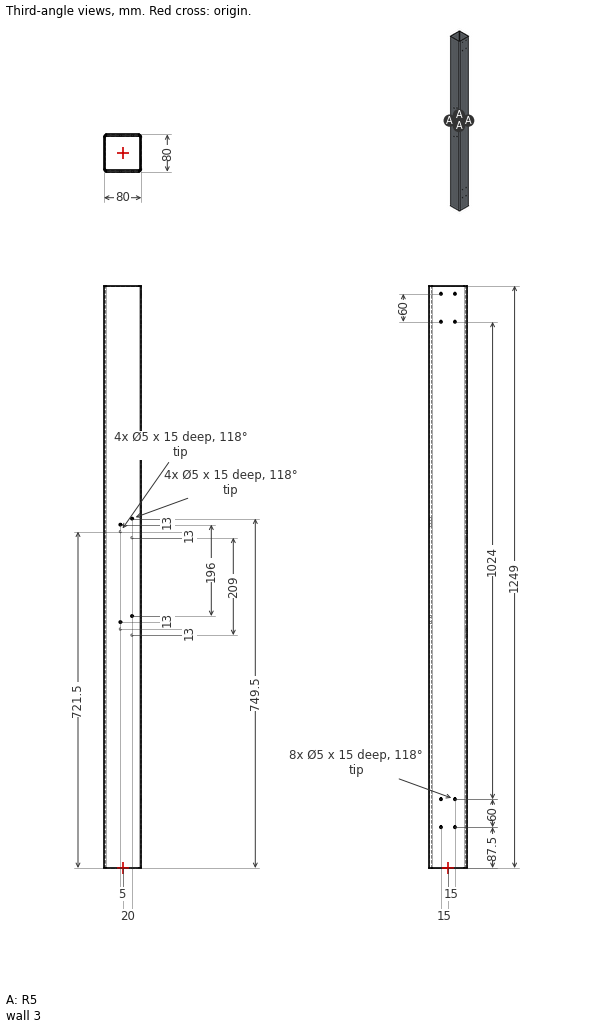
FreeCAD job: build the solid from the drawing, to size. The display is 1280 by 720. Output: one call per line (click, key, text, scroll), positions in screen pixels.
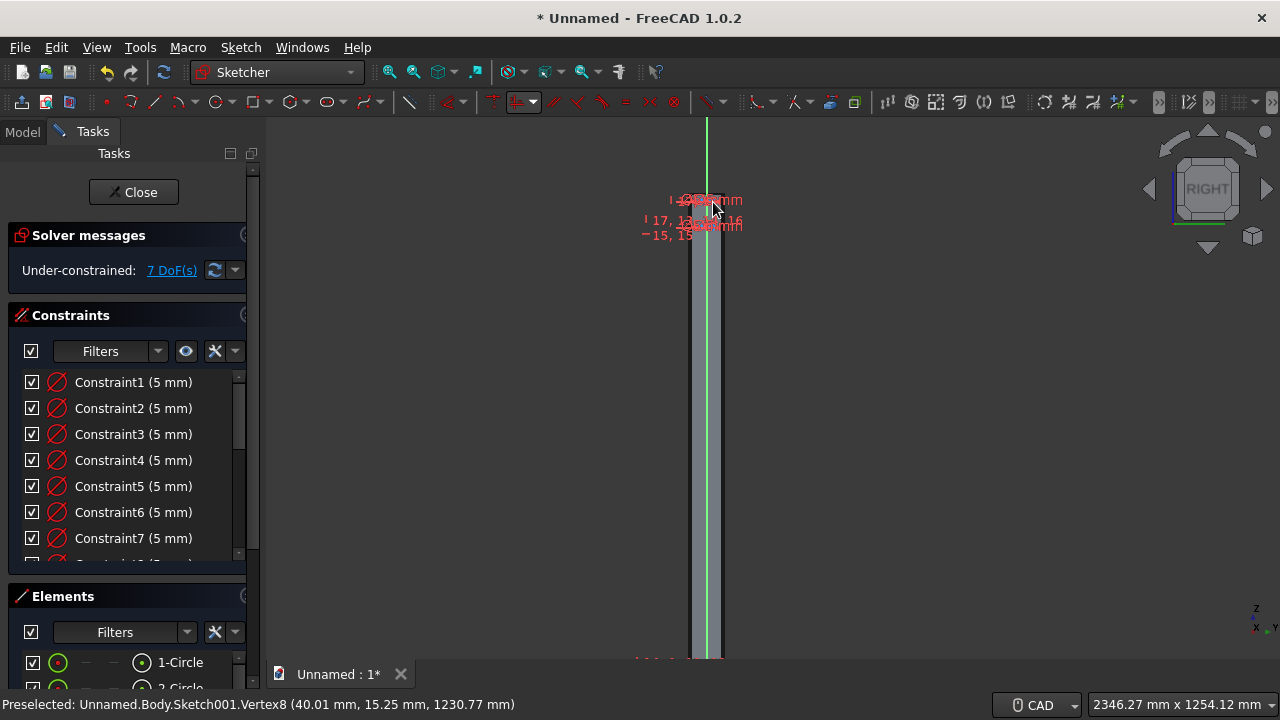
scroll(700, 202, up, 4)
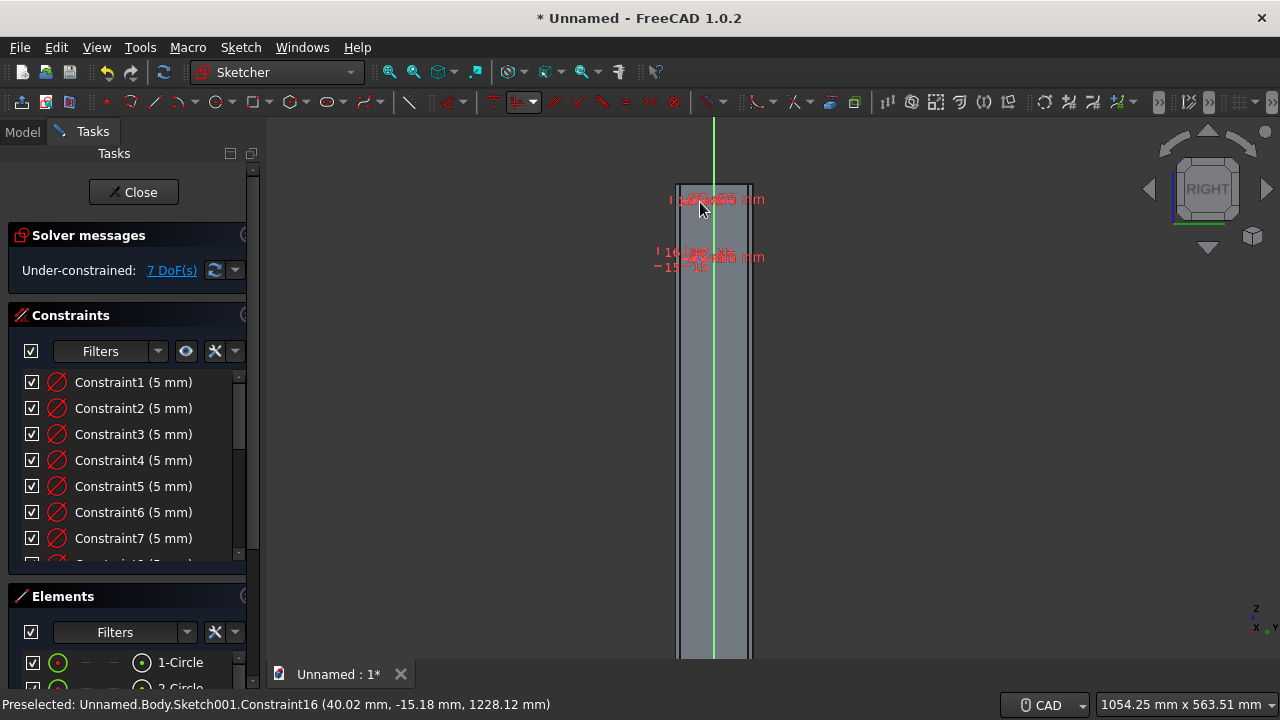
scroll(700, 201, up, 4)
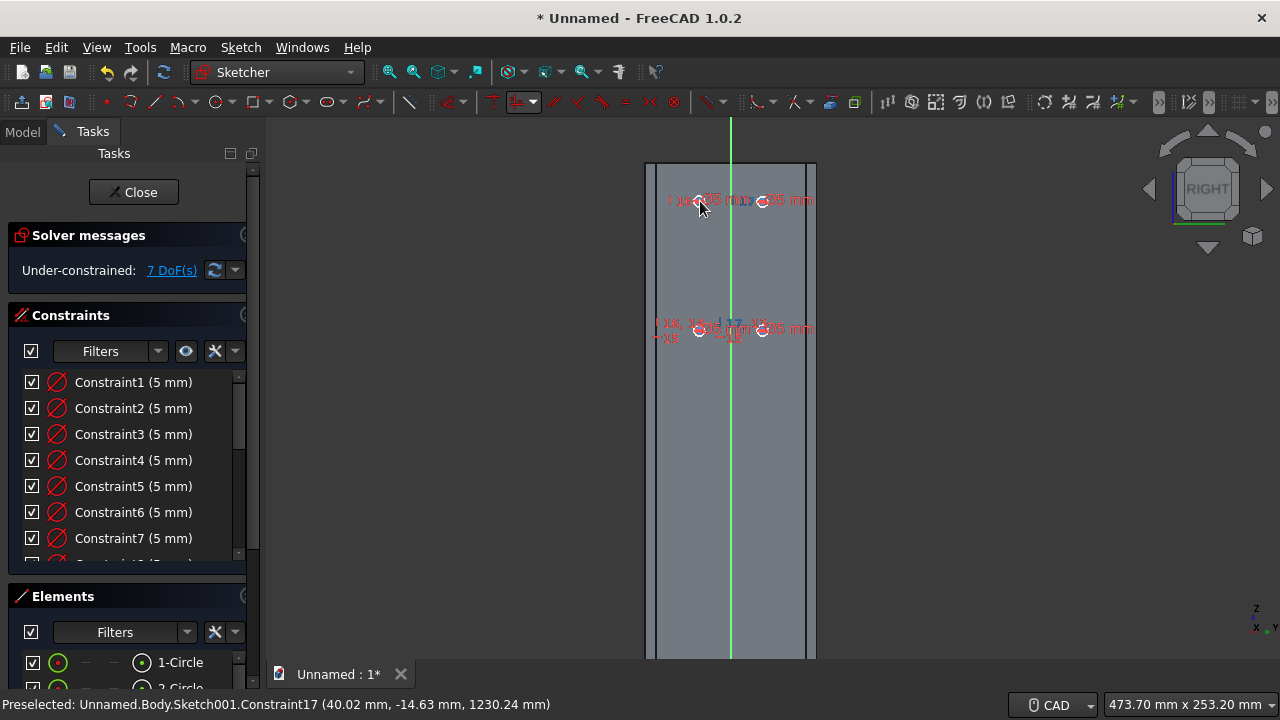
click(699, 201)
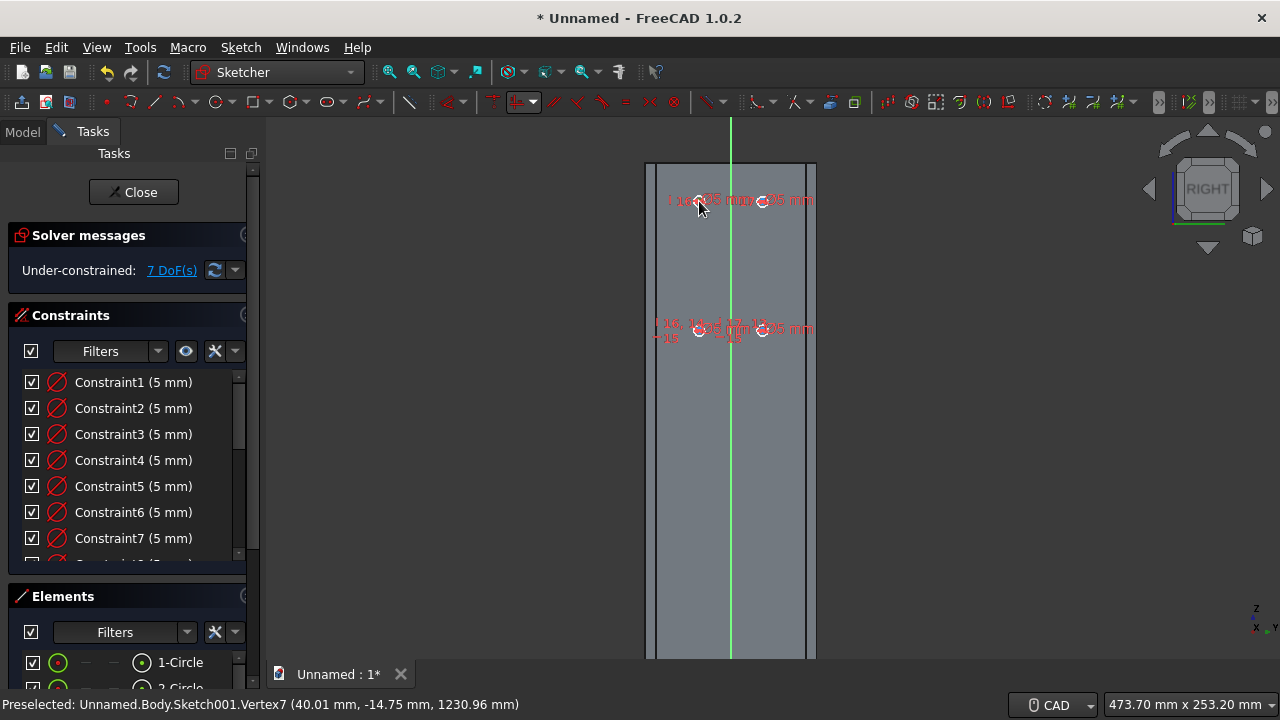
scroll(700, 211, down, 10)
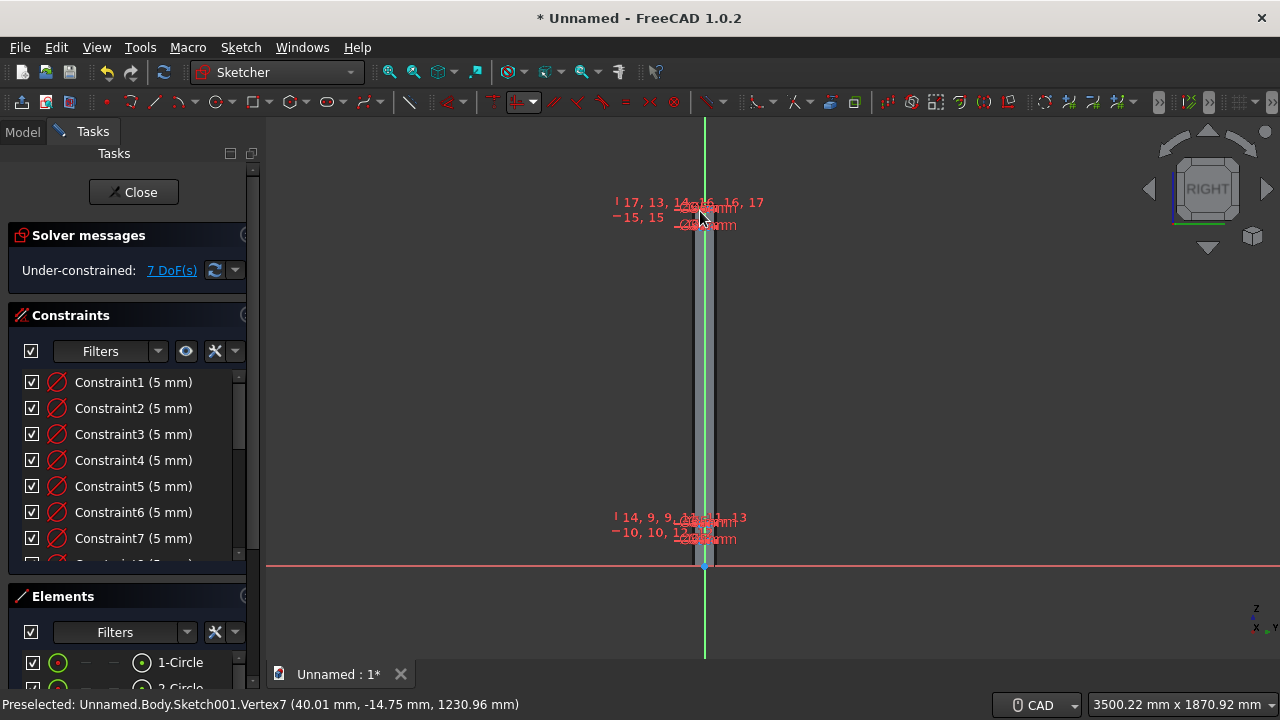
scroll(709, 210, up, 2)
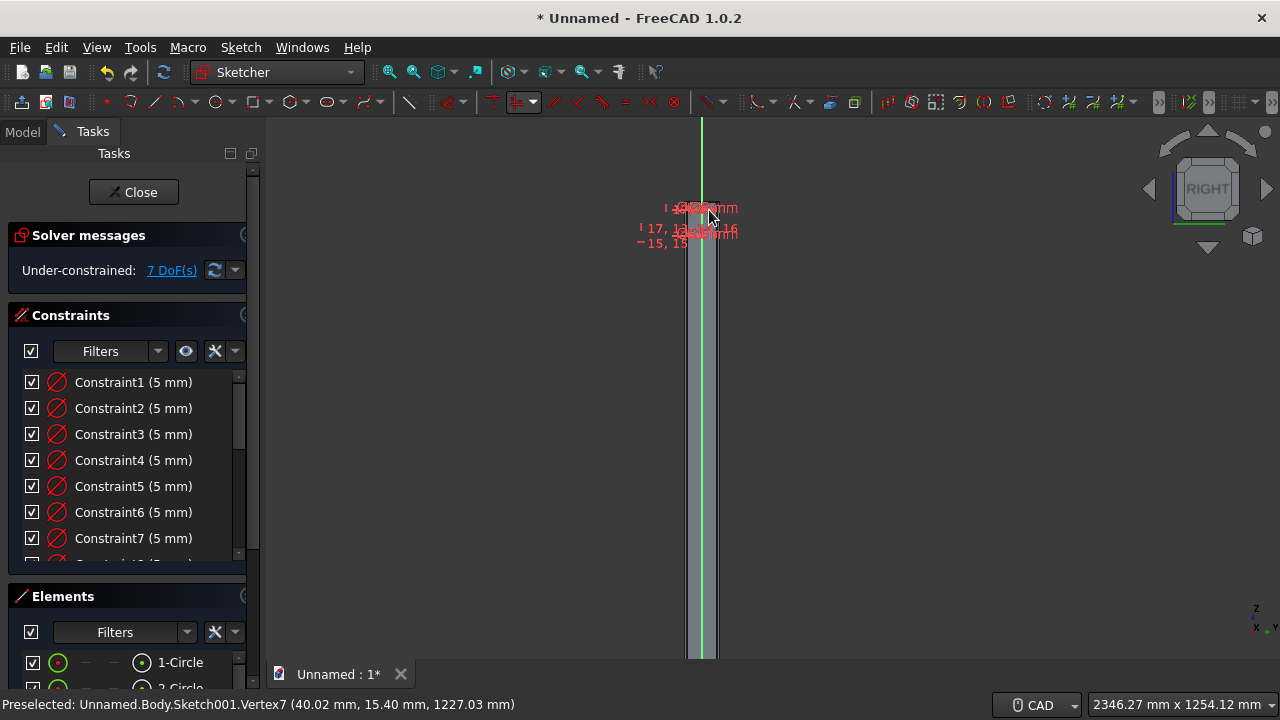
scroll(709, 210, up, 4)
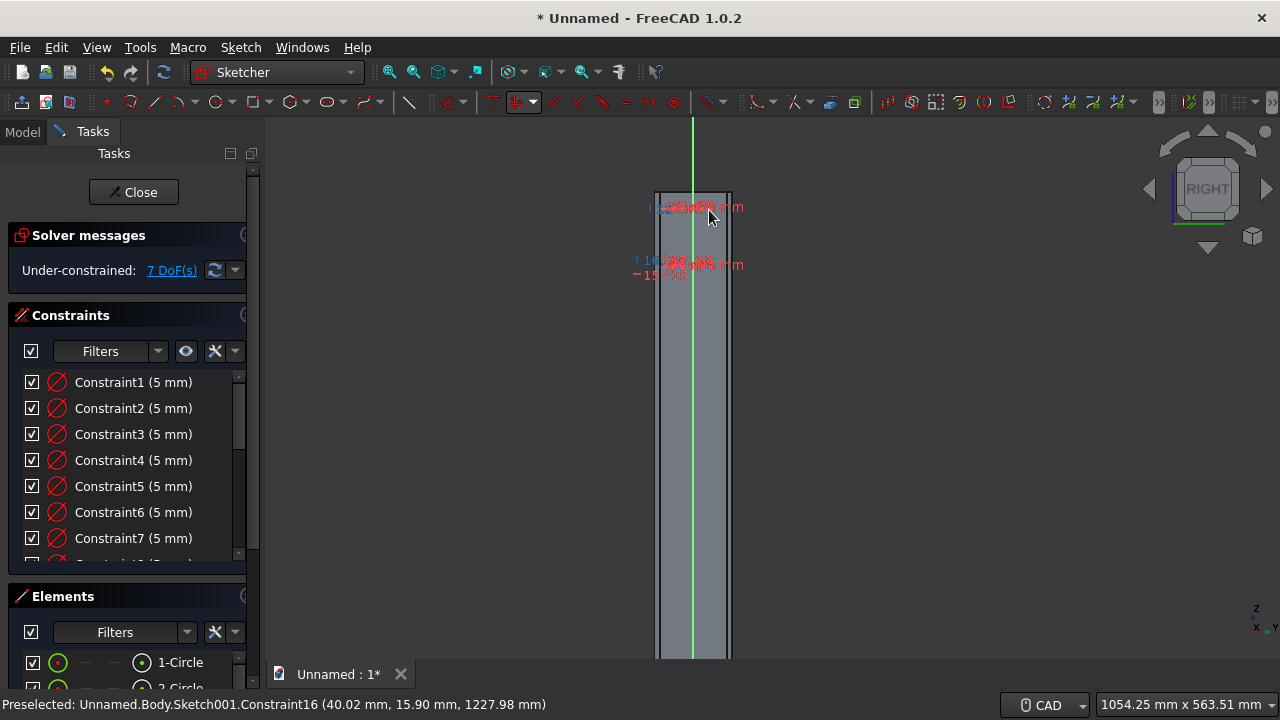
click(707, 209)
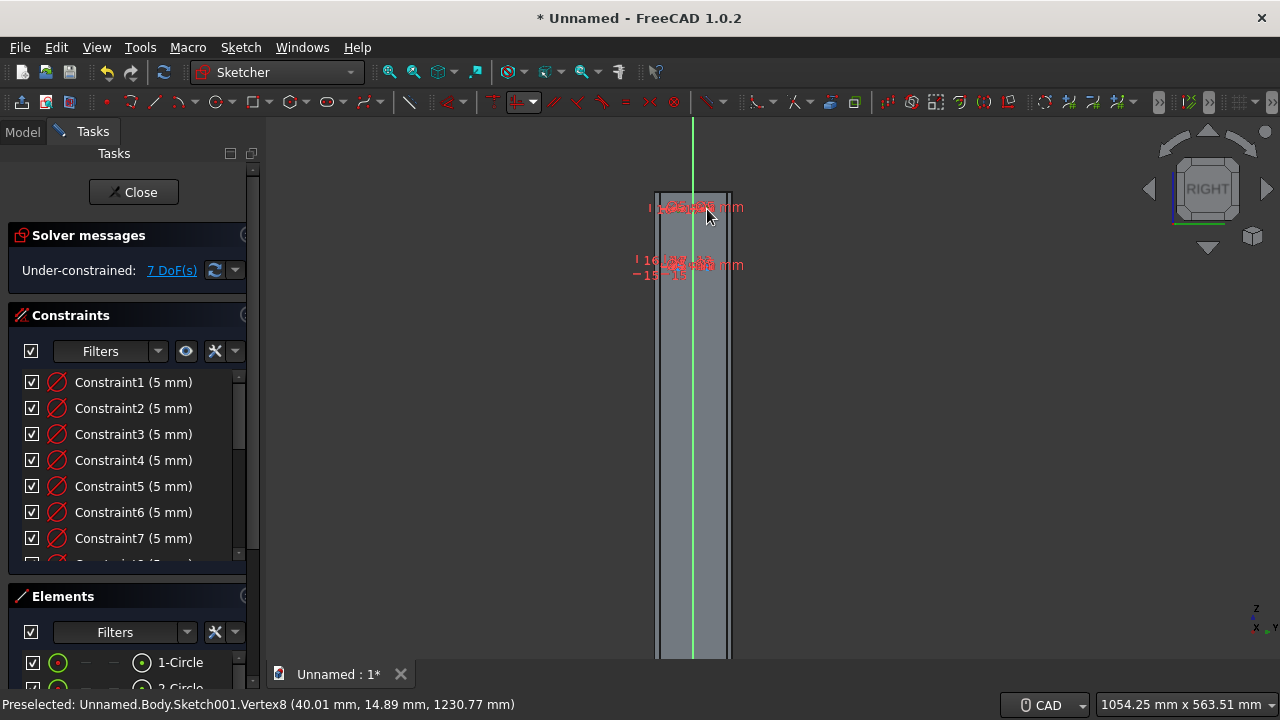
key(h)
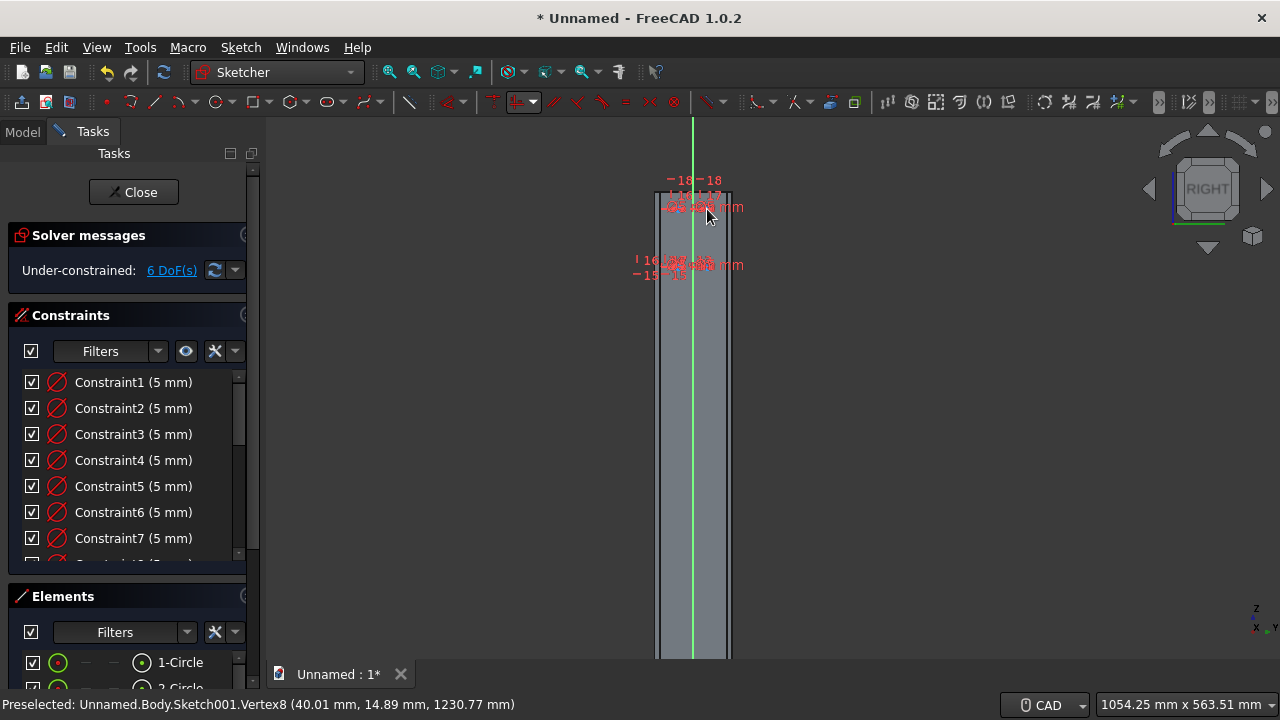
key(d)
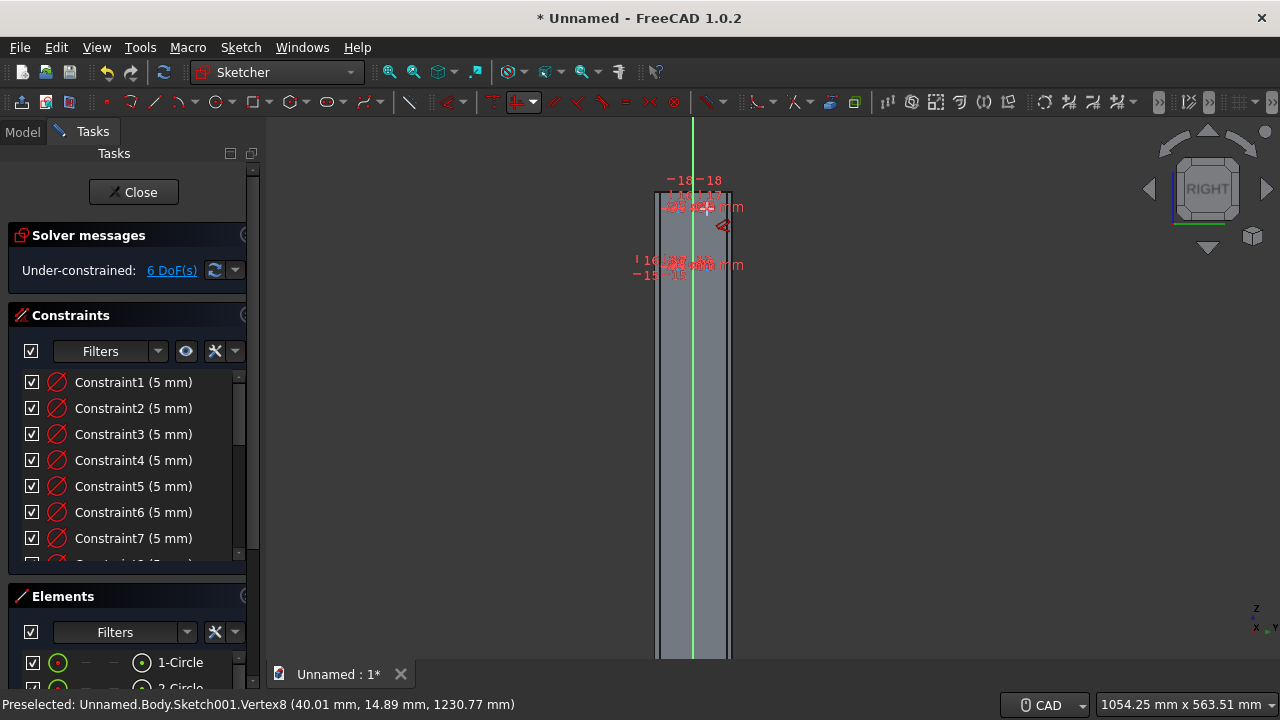
scroll(709, 211, down, 6)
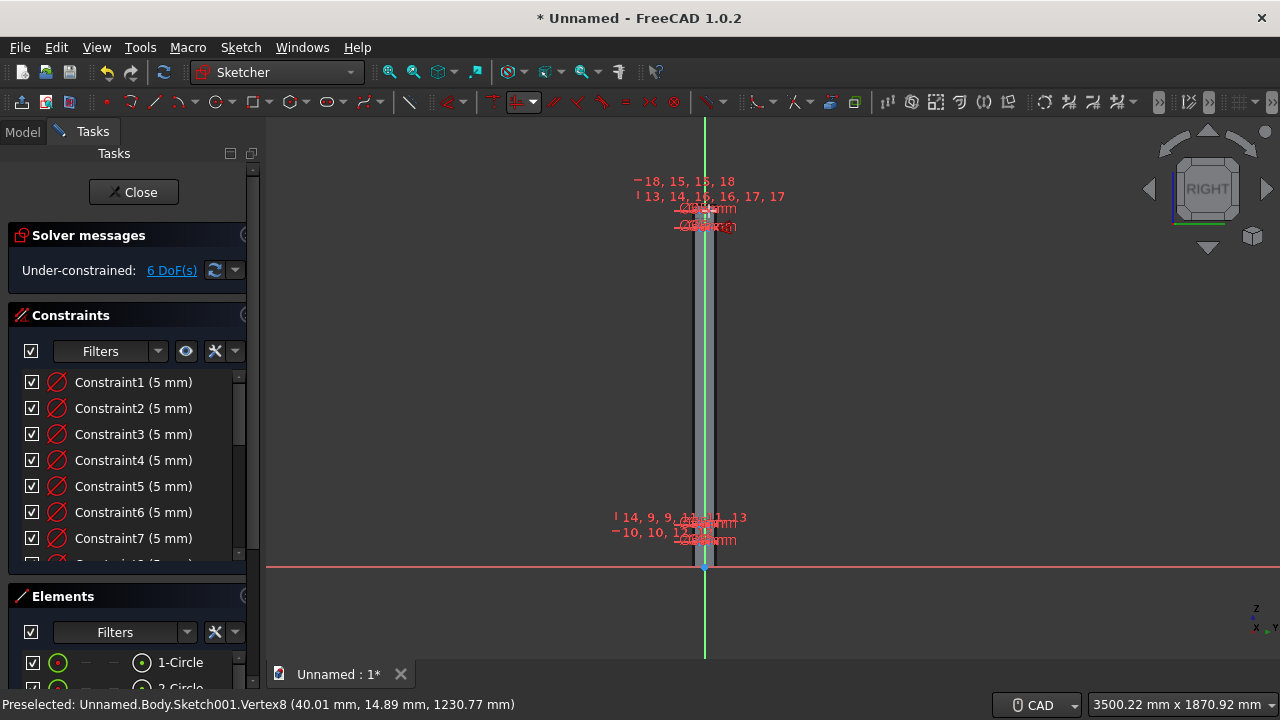
scroll(709, 525, up, 12)